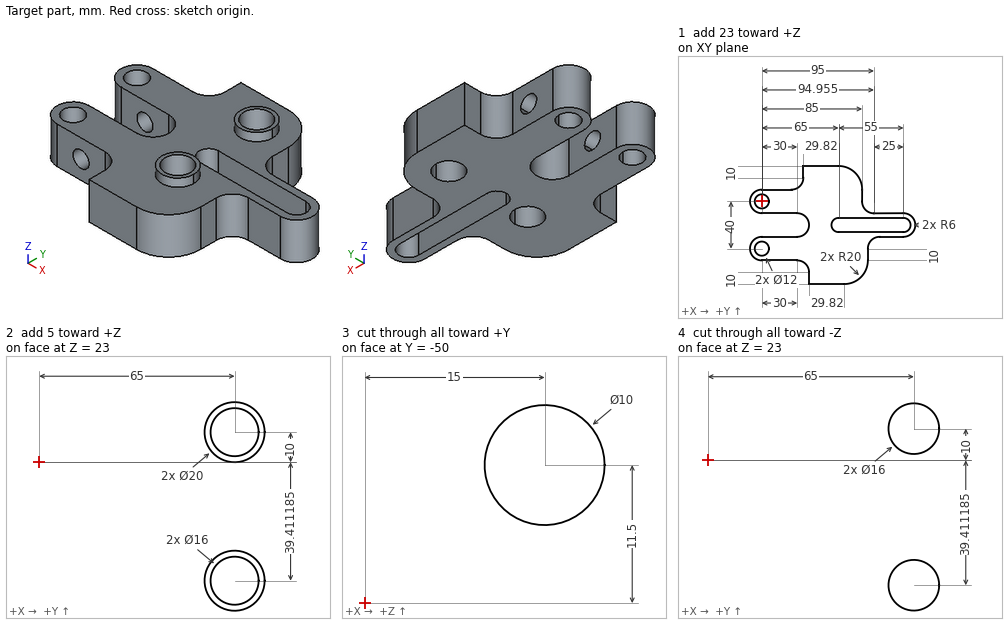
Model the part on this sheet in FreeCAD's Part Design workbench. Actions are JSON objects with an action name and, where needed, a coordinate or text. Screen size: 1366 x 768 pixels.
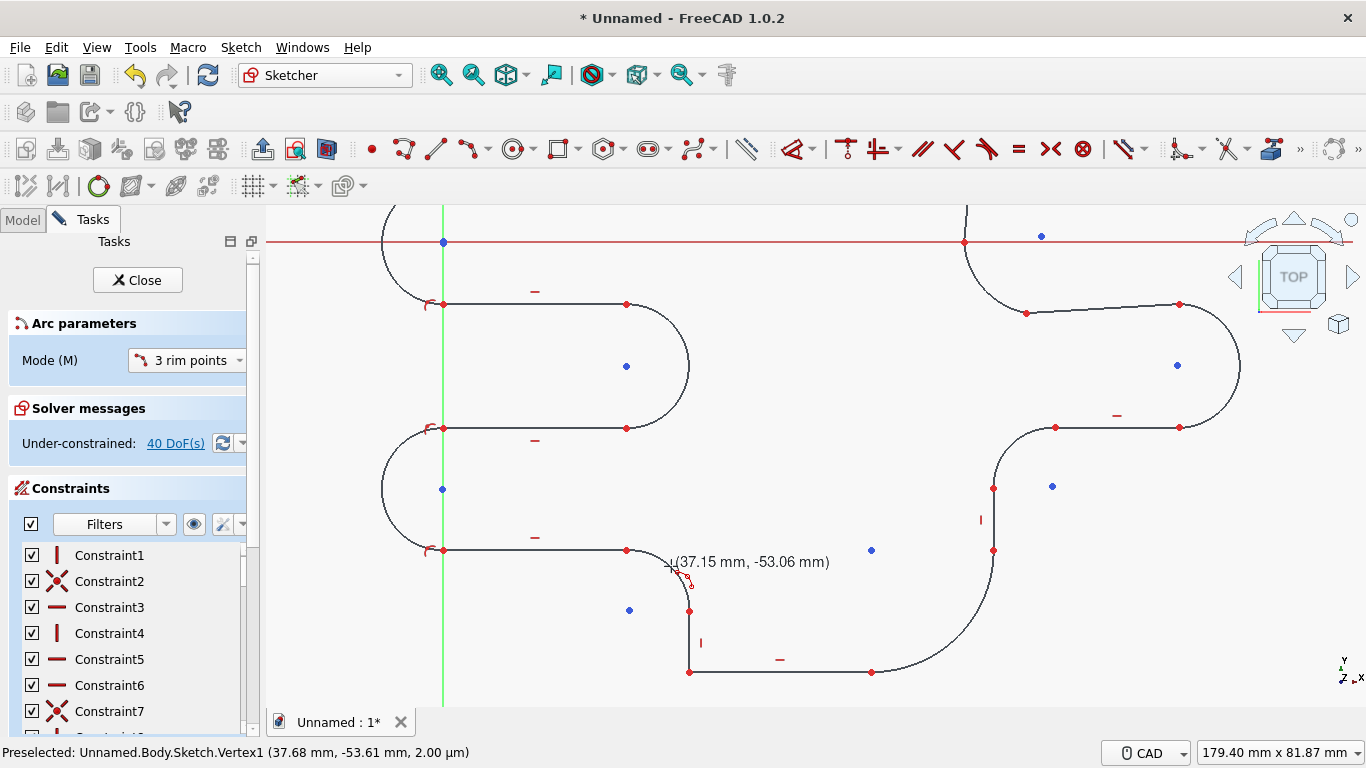
{"action": "left_click", "coordinate": [648, 150]}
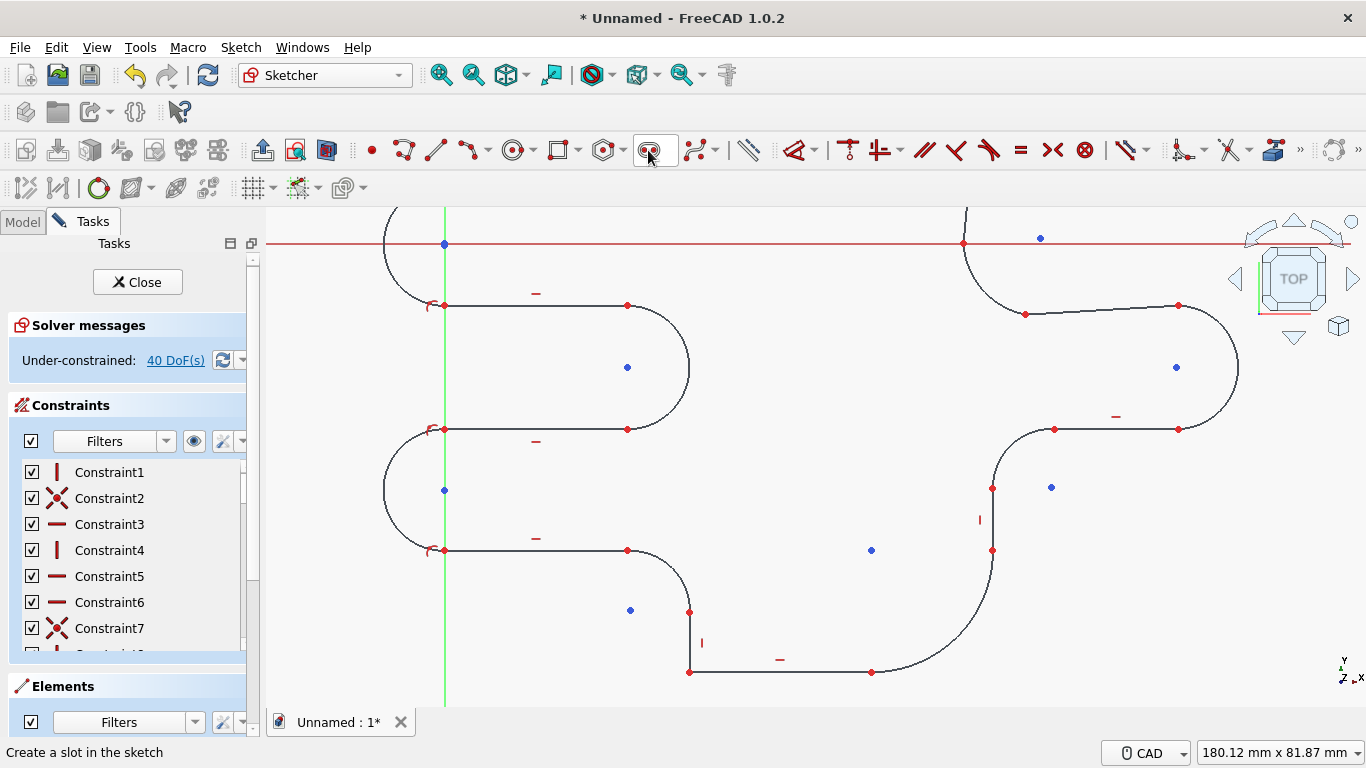
{"action": "left_click", "coordinate": [842, 366]}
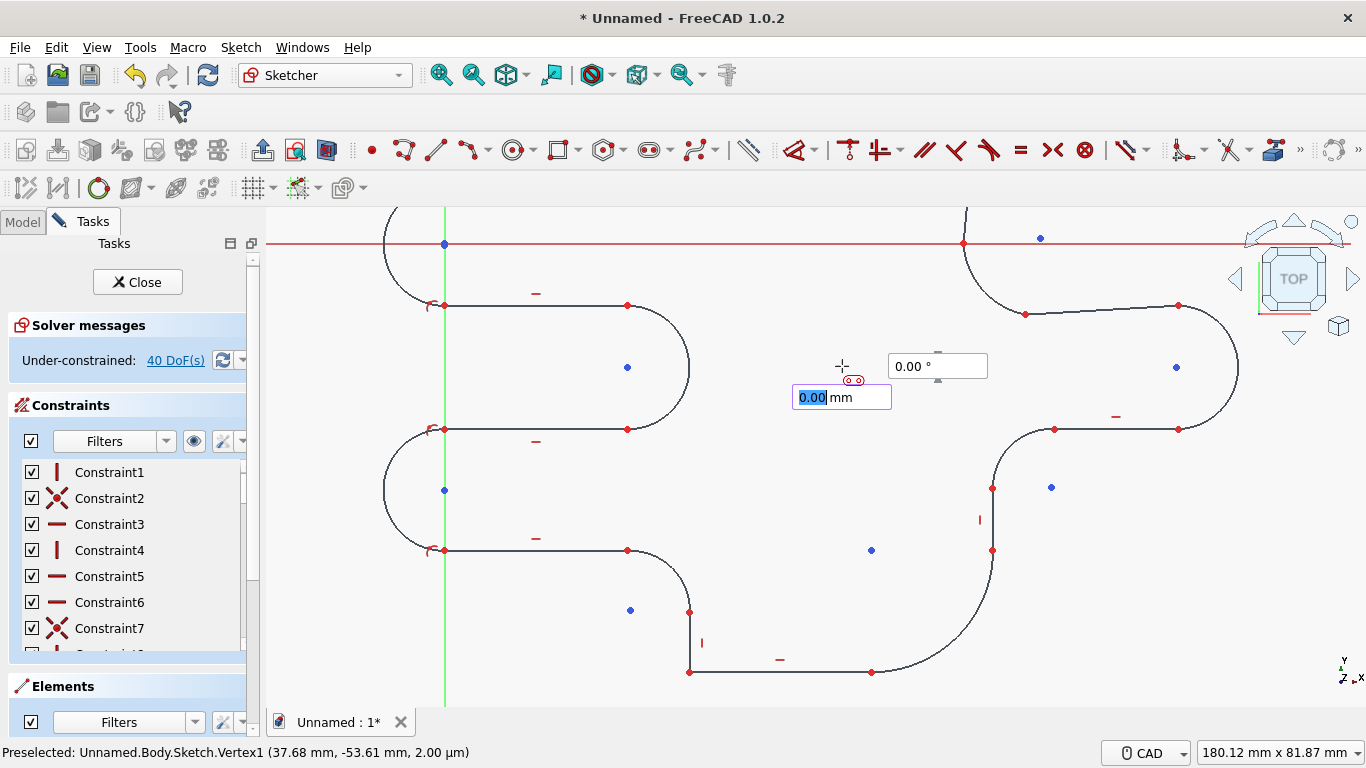
{"action": "left_click", "coordinate": [1178, 366]}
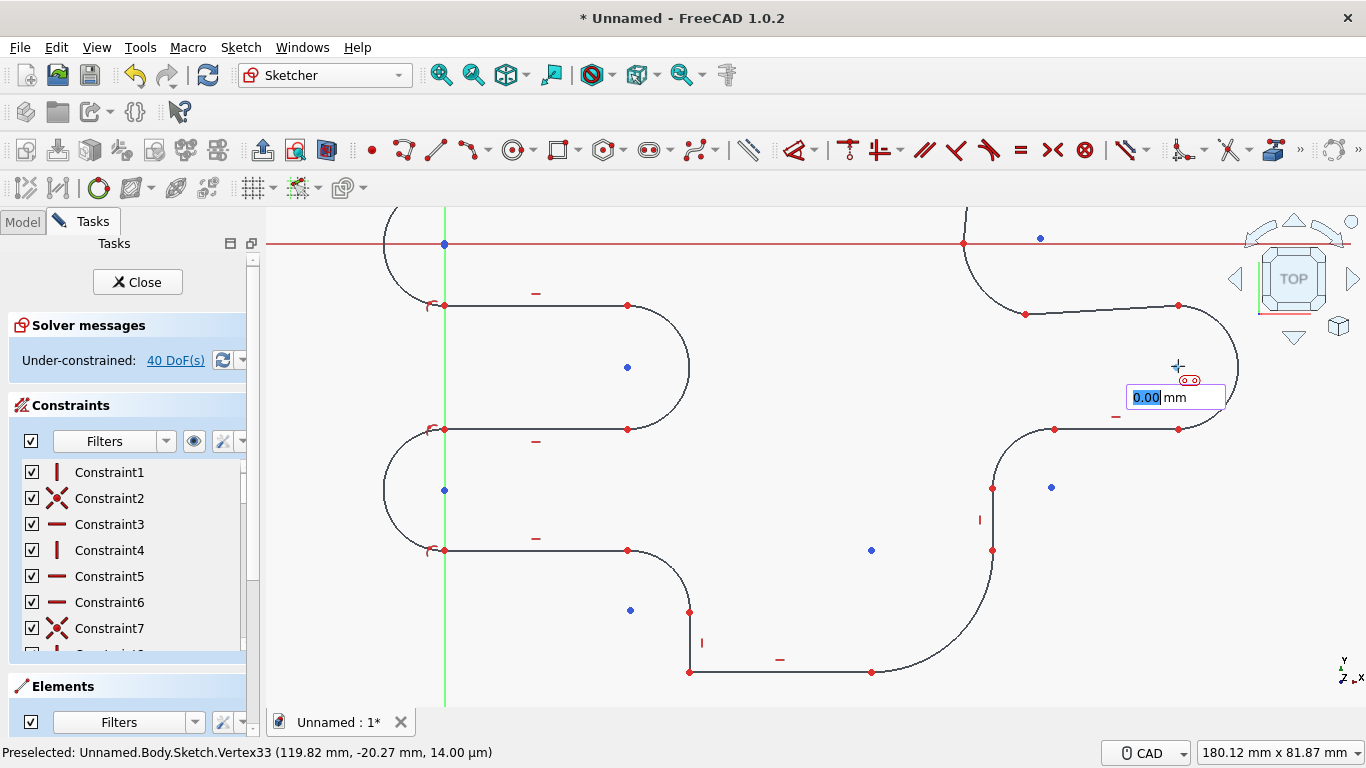
{"action": "left_click", "coordinate": [1010, 402]}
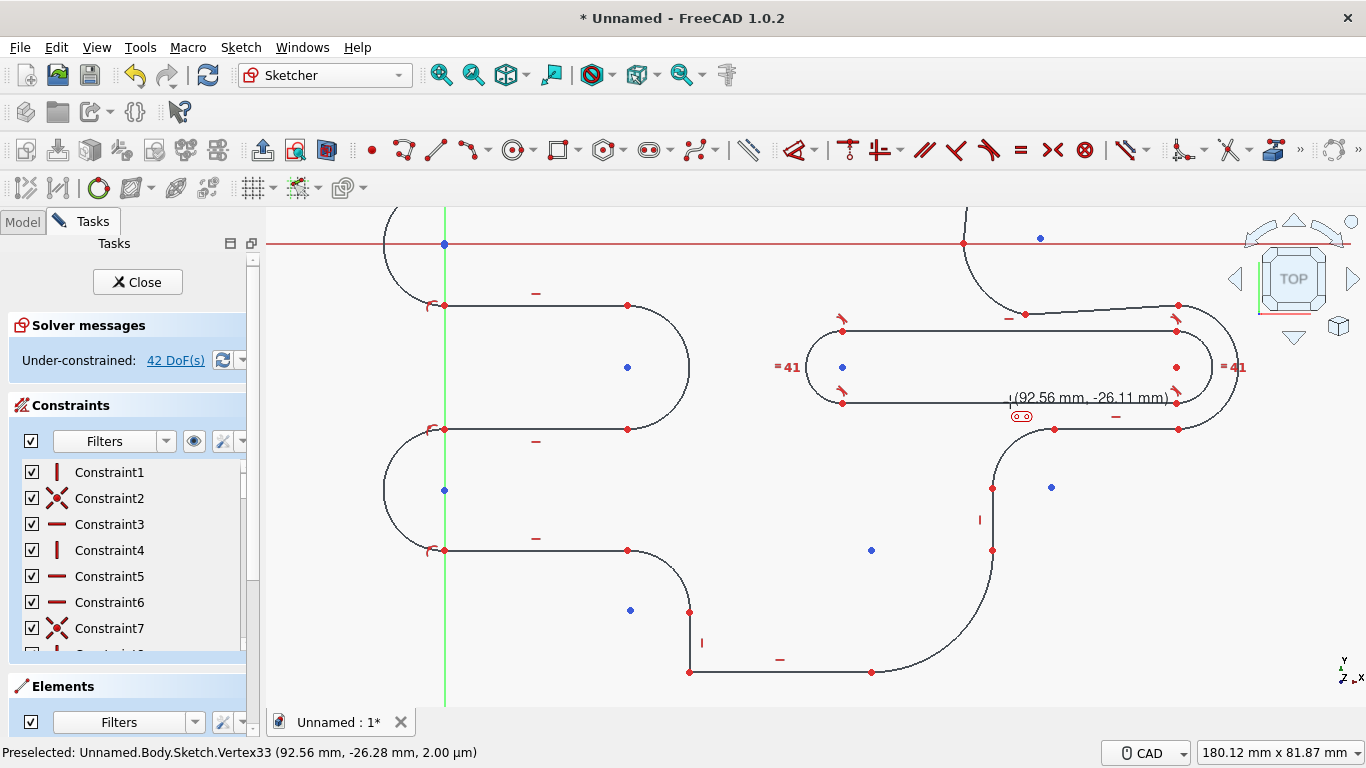
{"action": "left_click", "coordinate": [514, 150]}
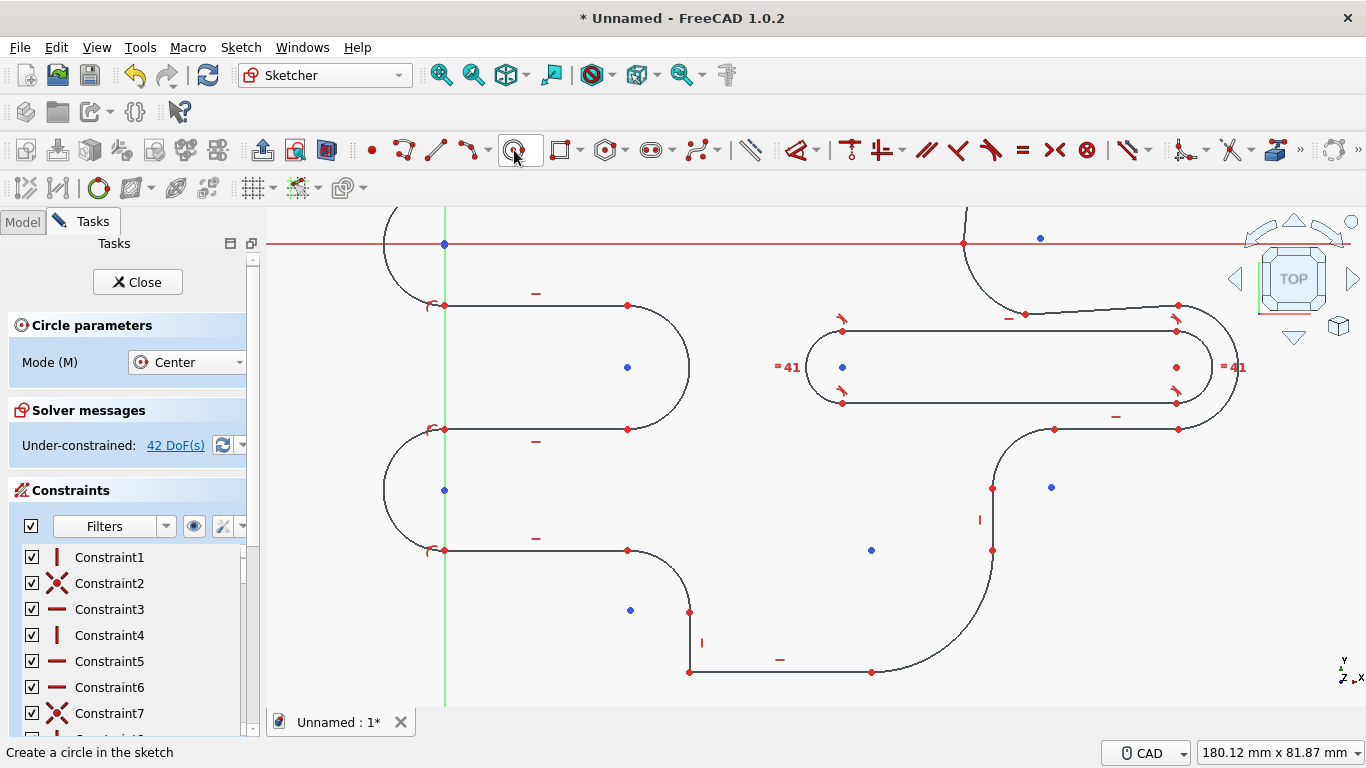
{"action": "left_click", "coordinate": [445, 488]}
{"action": "mouse_move", "coordinate": [471, 462]}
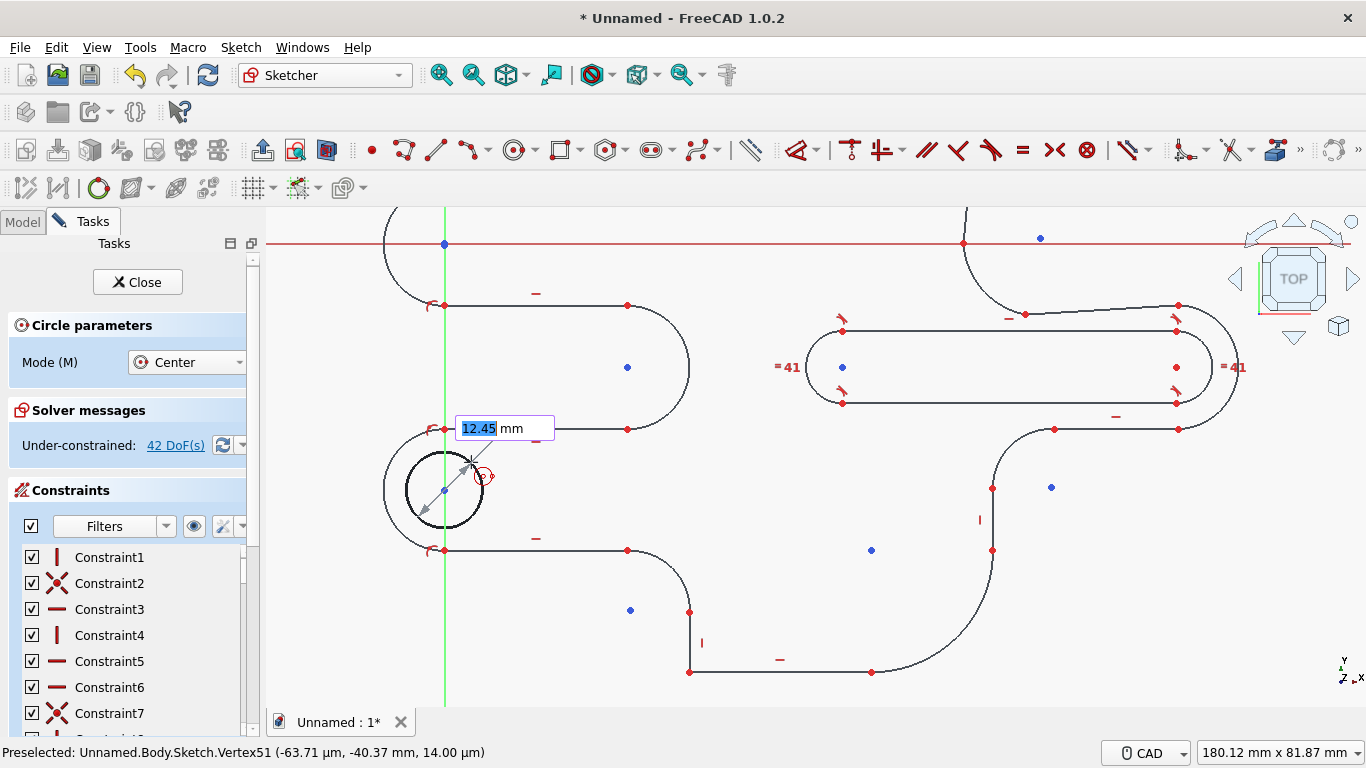
{"action": "type", "text": "12"}
{"action": "key", "text": "Return"}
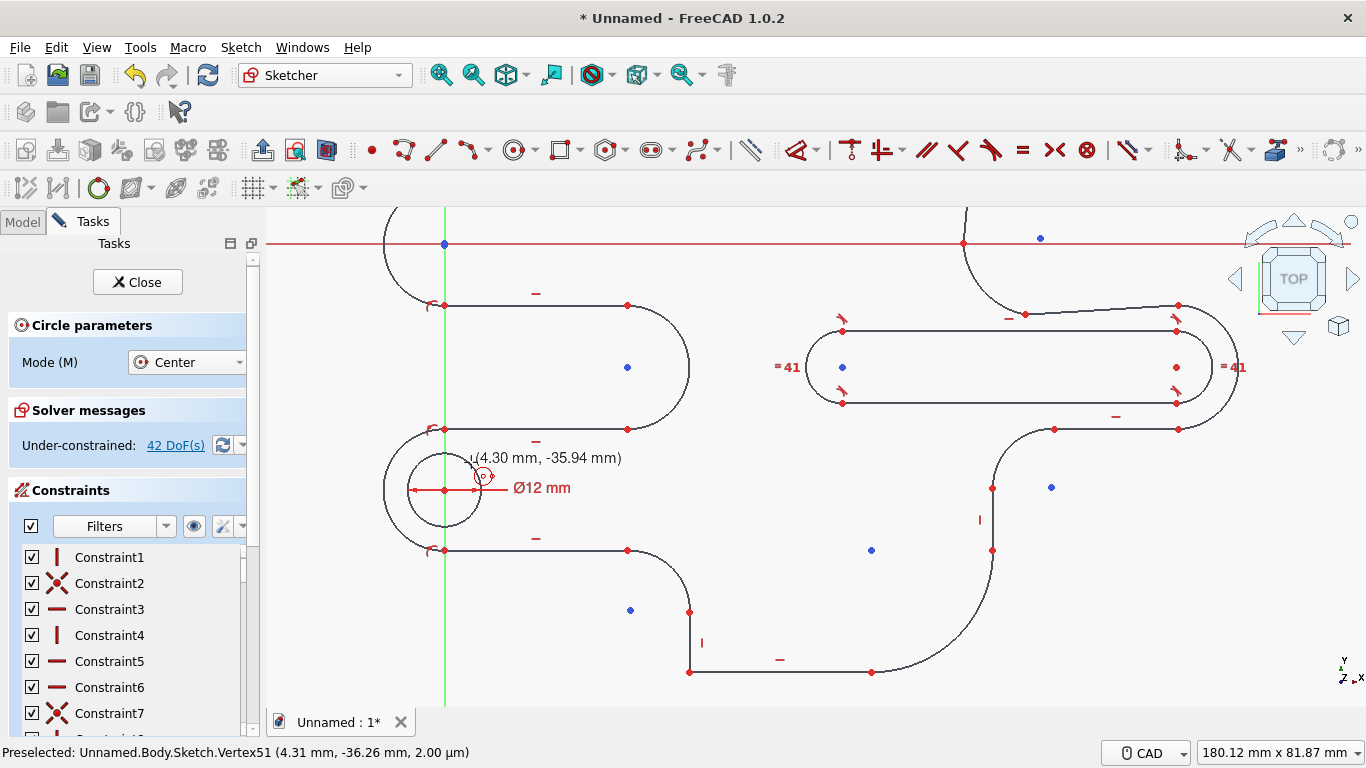
{"action": "left_click", "coordinate": [445, 244]}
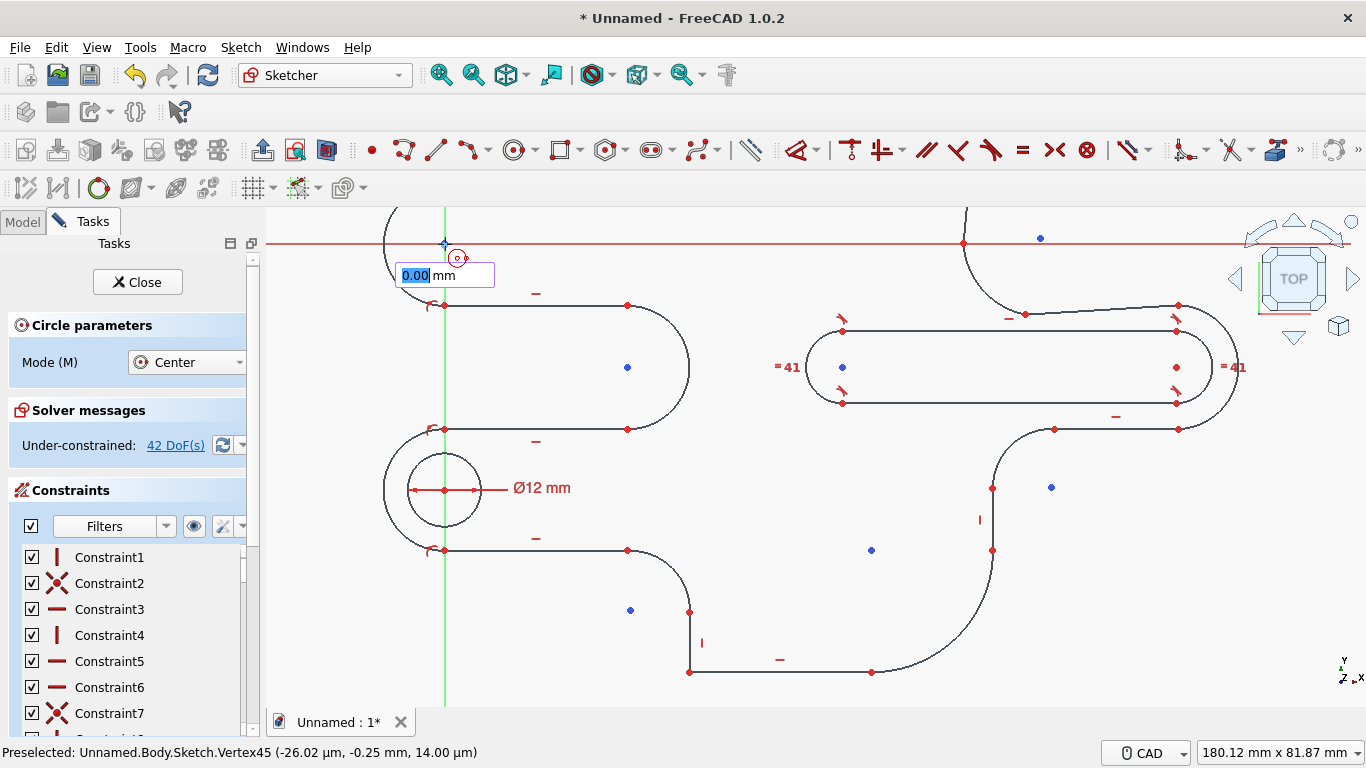
{"action": "scroll", "coordinate": [670, 568], "scroll_direction": "down", "scroll_amount": 3}
{"action": "mouse_move", "coordinate": [561, 376]}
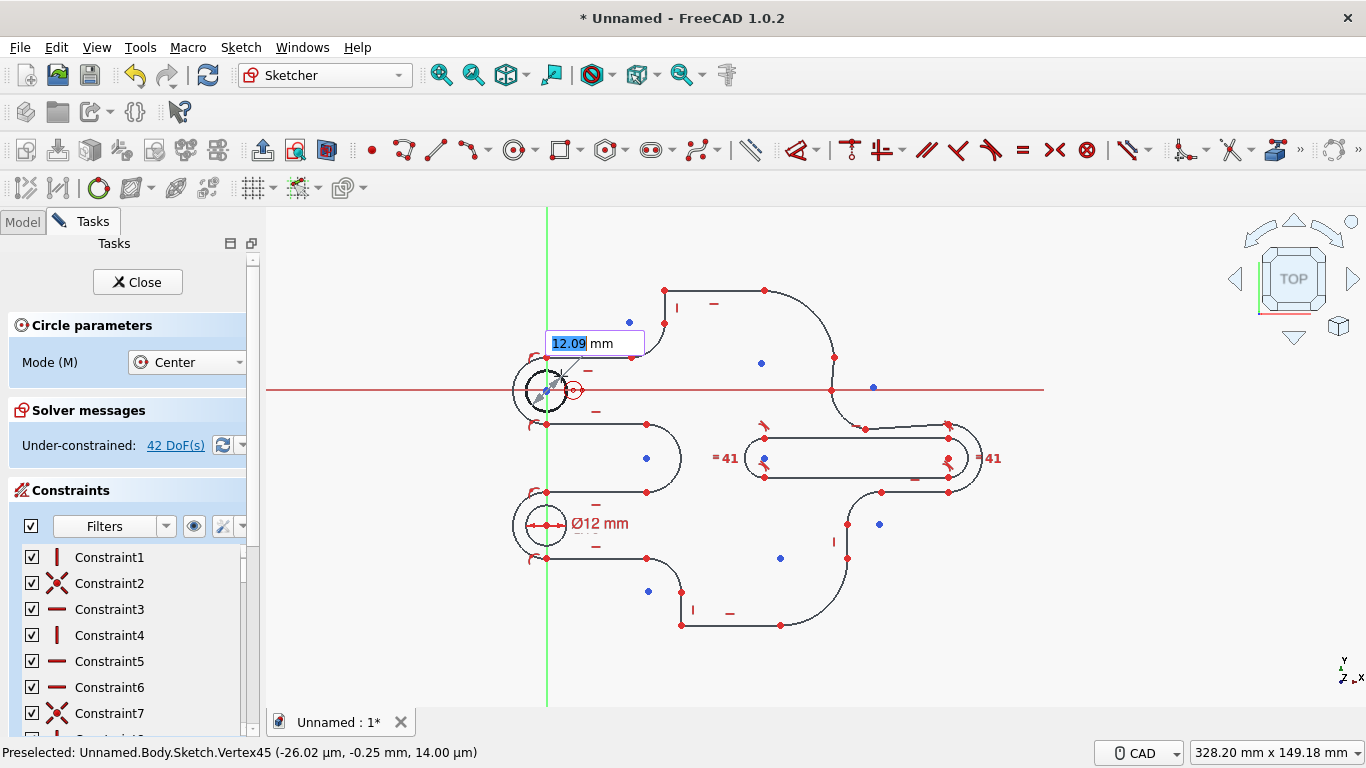
{"action": "type", "text": "12"}
{"action": "key", "text": "Return"}
{"action": "key", "text": "Escape"}